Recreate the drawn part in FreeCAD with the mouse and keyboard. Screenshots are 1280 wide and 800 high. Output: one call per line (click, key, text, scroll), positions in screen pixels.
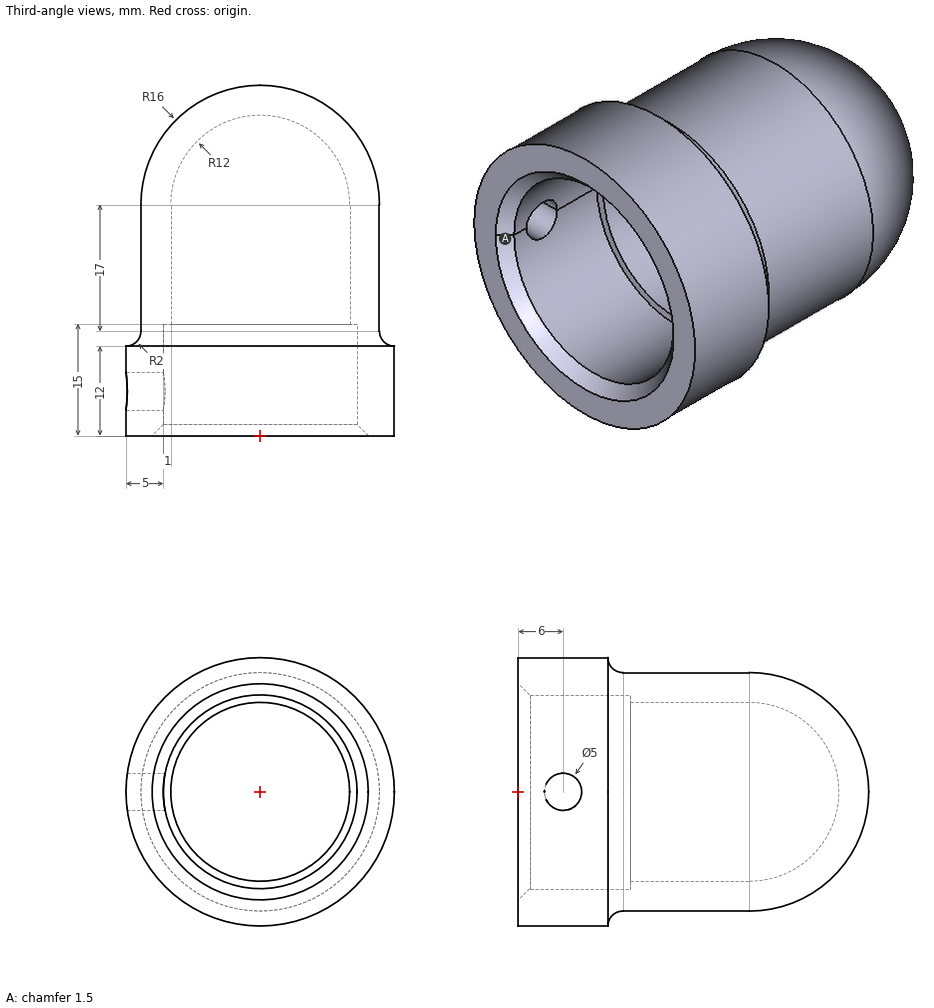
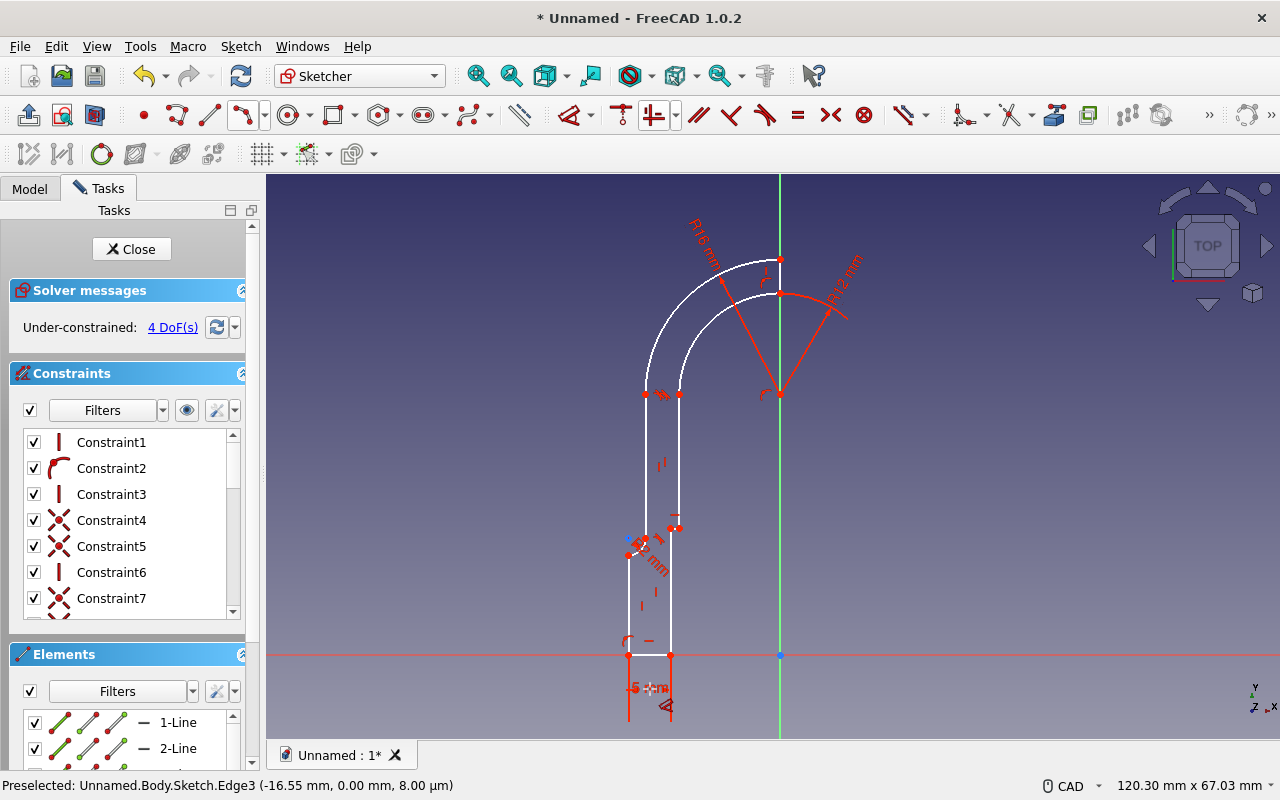
scroll(675, 529, up, 8)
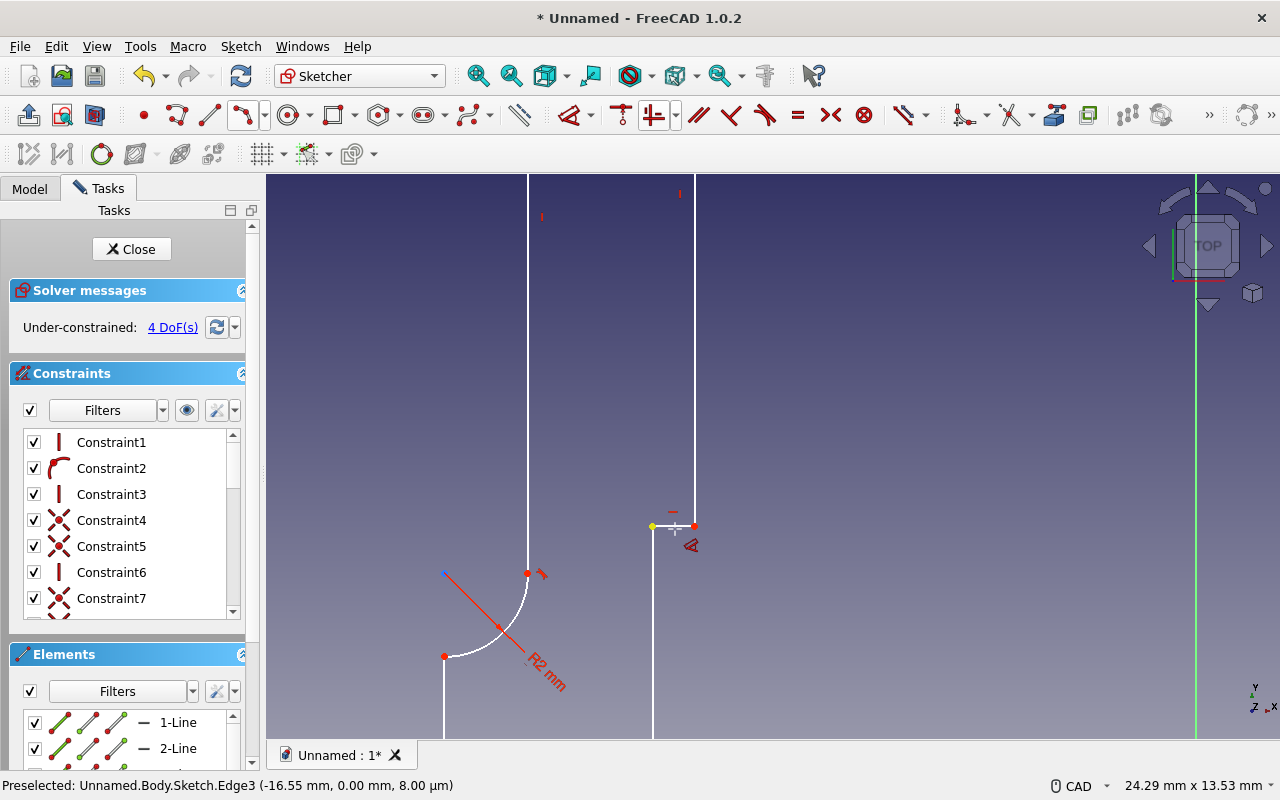
click(674, 526)
click(674, 560)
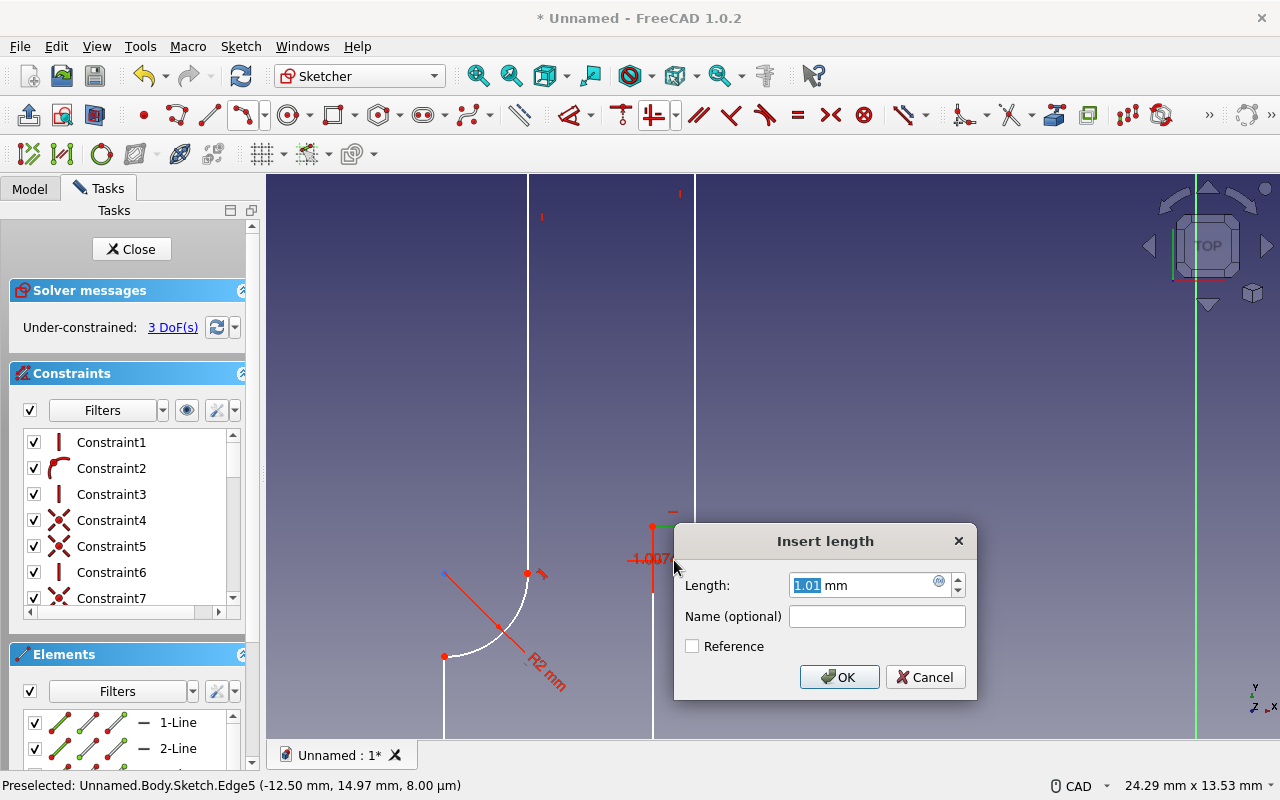
text(1)
key(Return)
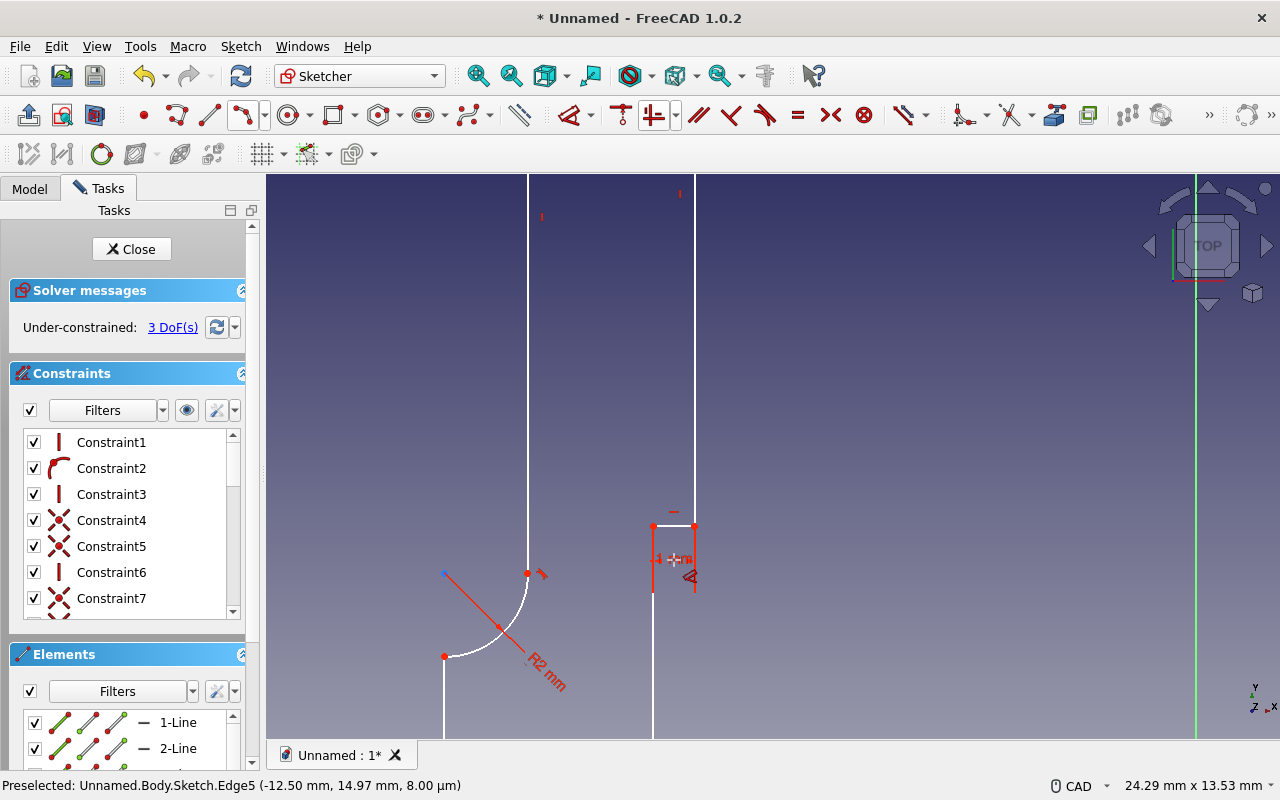
scroll(675, 529, down, 8)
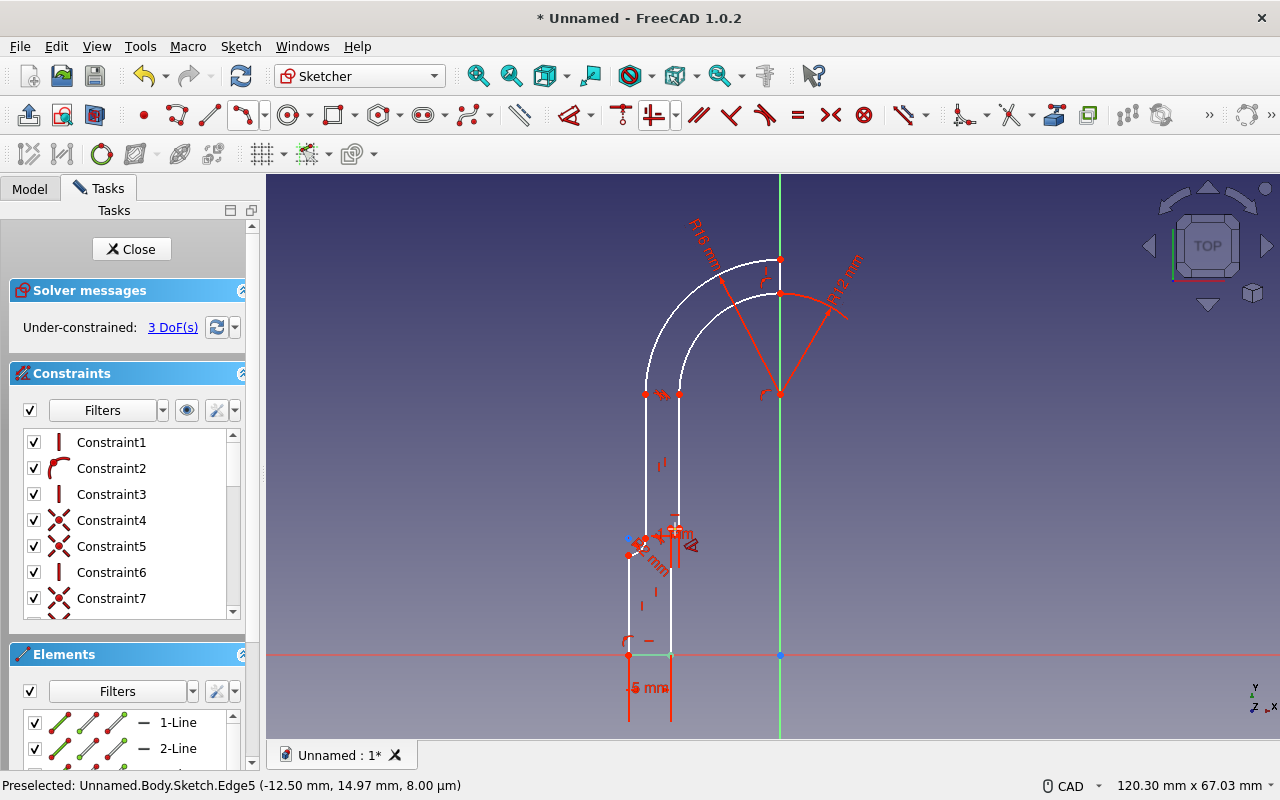
click(646, 495)
click(612, 467)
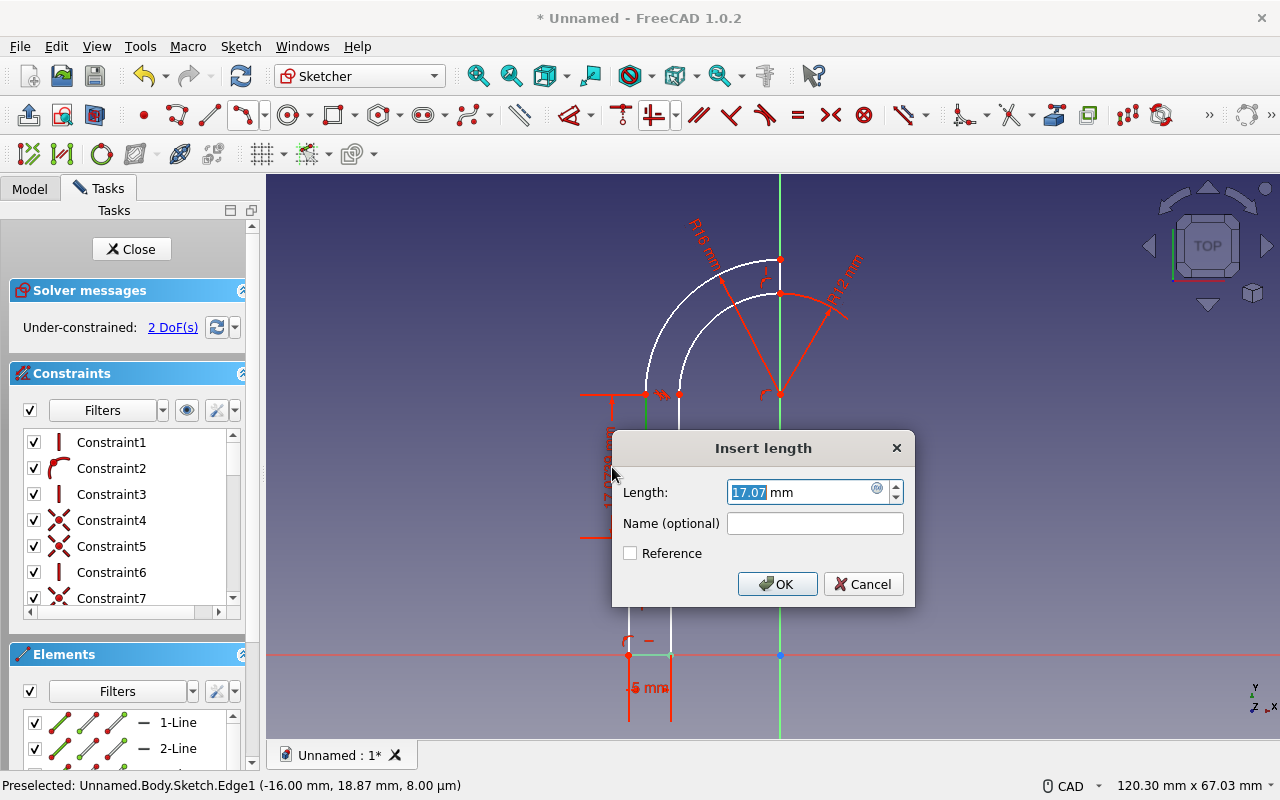
text(17)
key(Return)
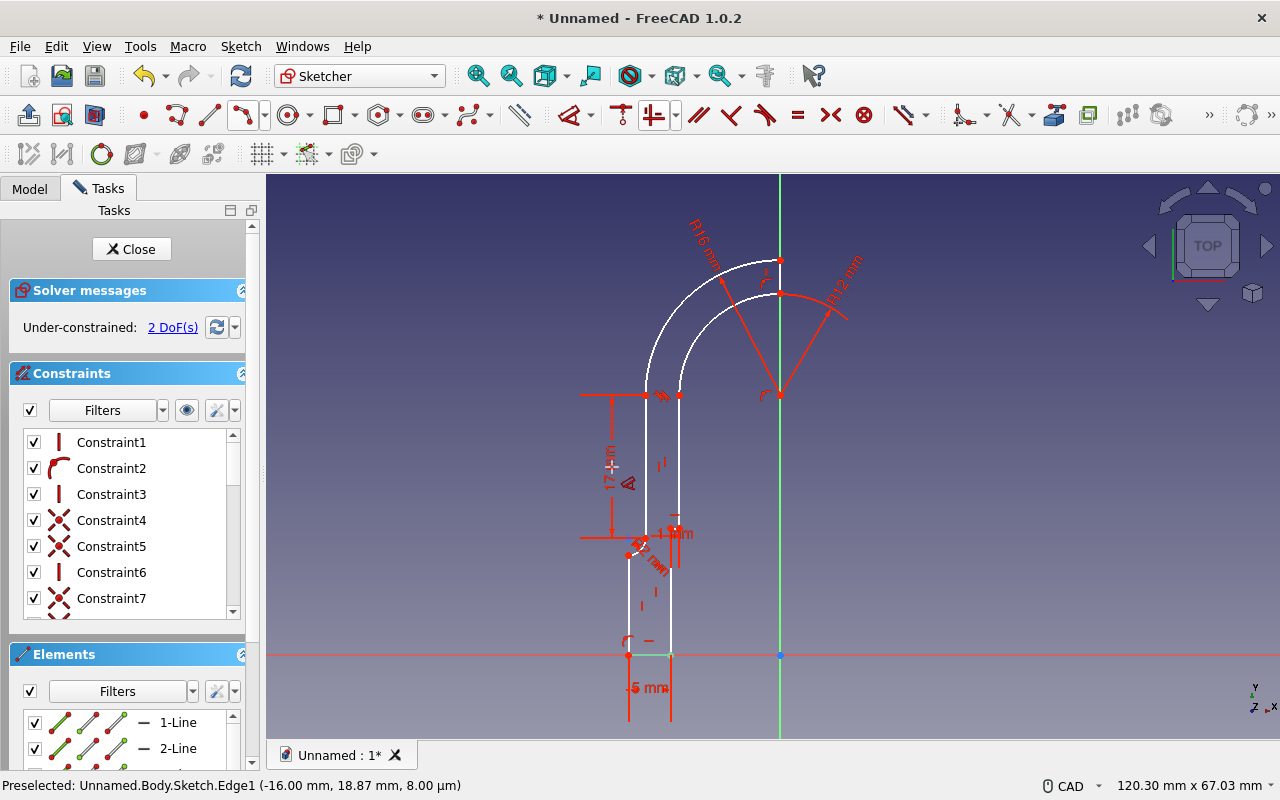
click(629, 585)
click(595, 605)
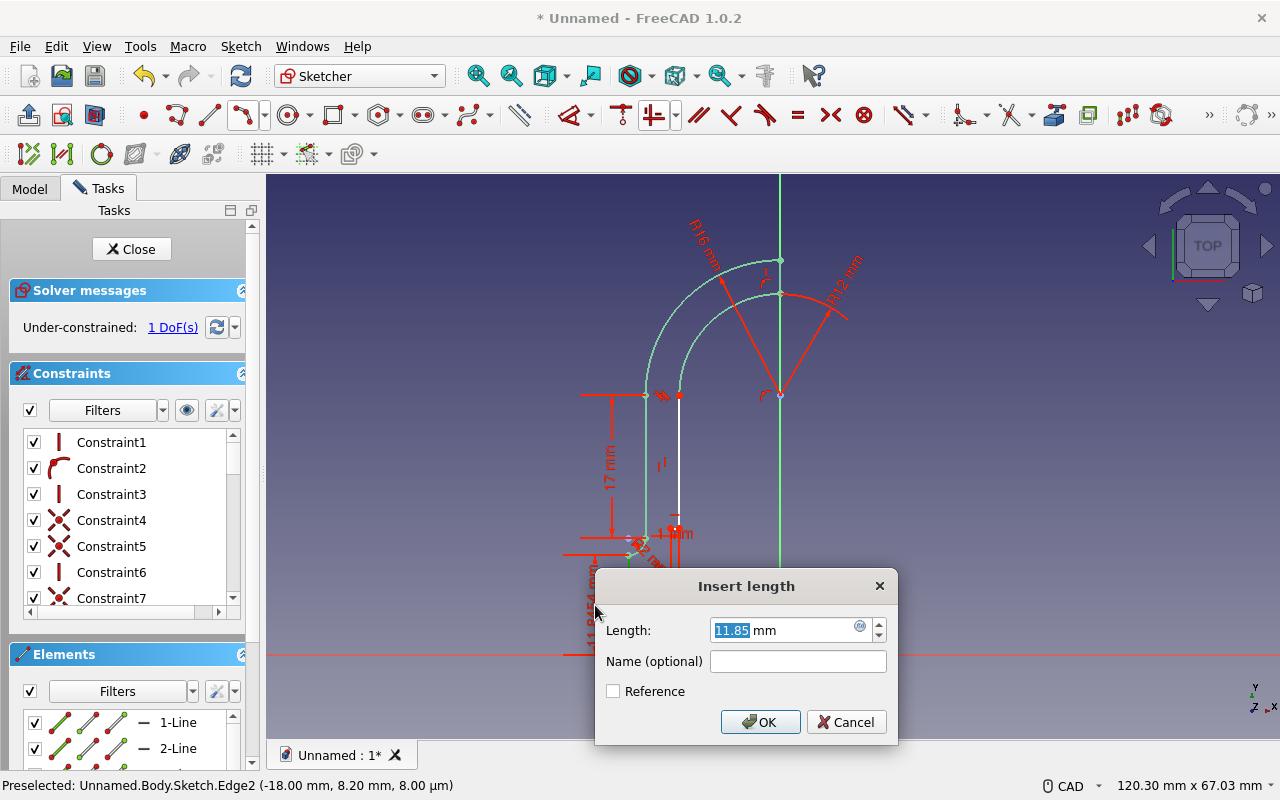
text(12)
key(Return)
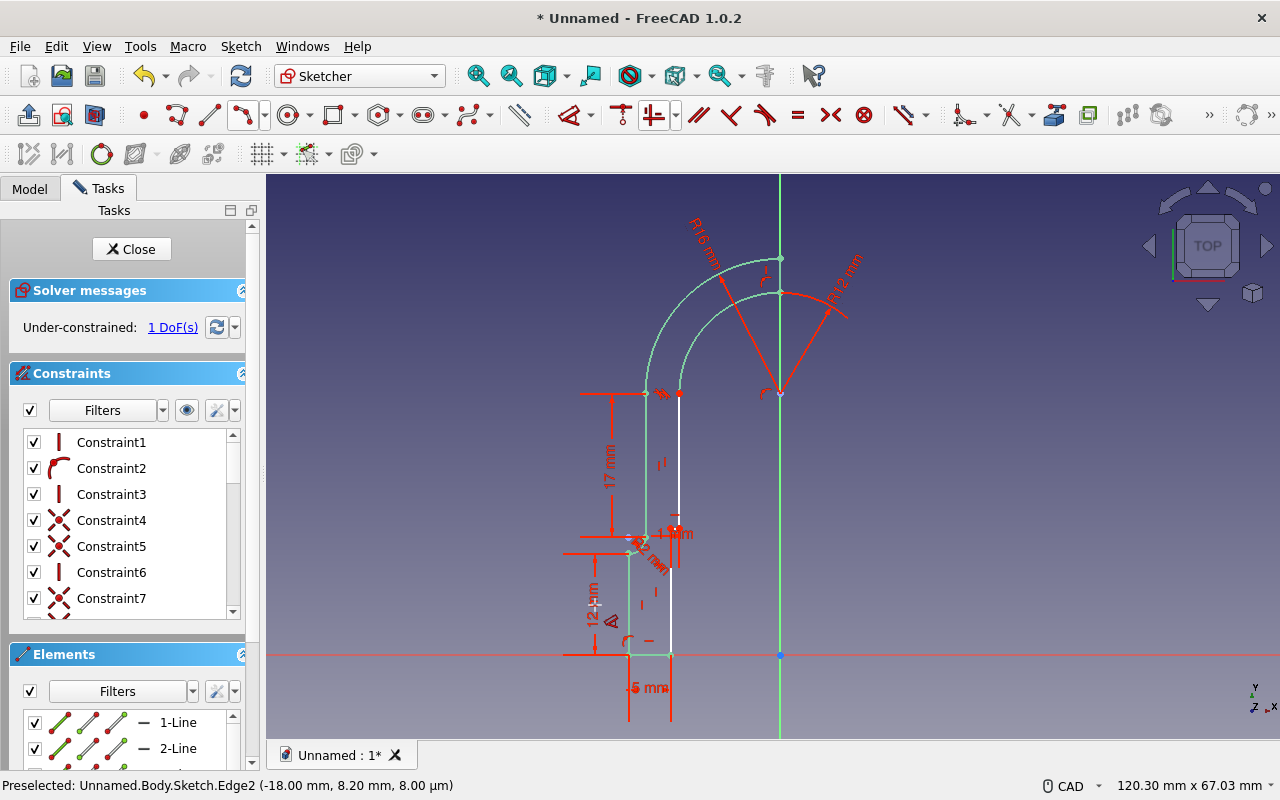
click(671, 617)
click(705, 592)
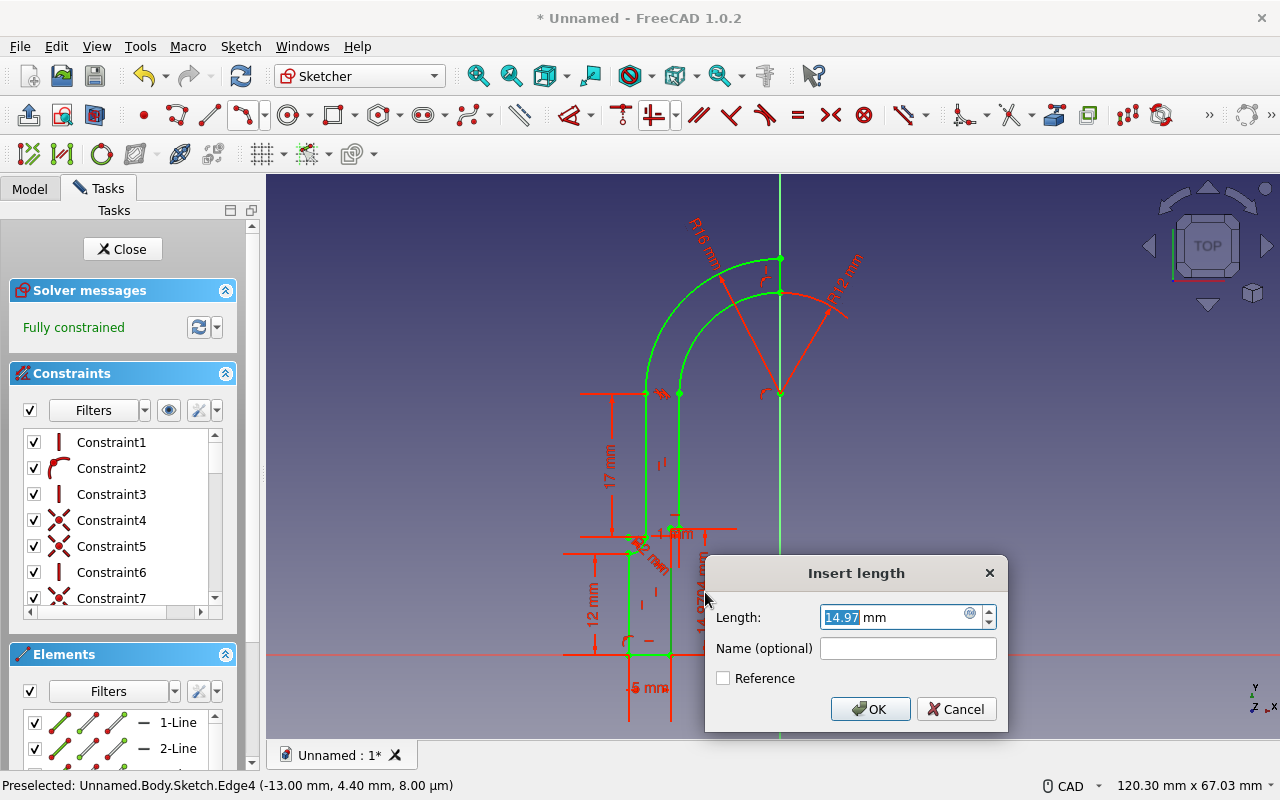
text(15)
key(Return)
key(Escape)